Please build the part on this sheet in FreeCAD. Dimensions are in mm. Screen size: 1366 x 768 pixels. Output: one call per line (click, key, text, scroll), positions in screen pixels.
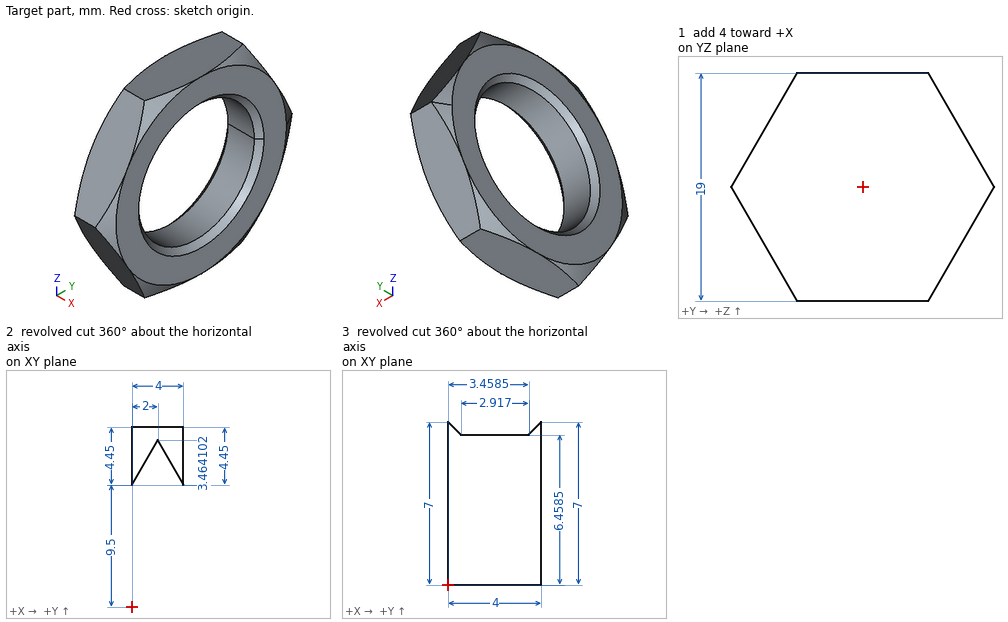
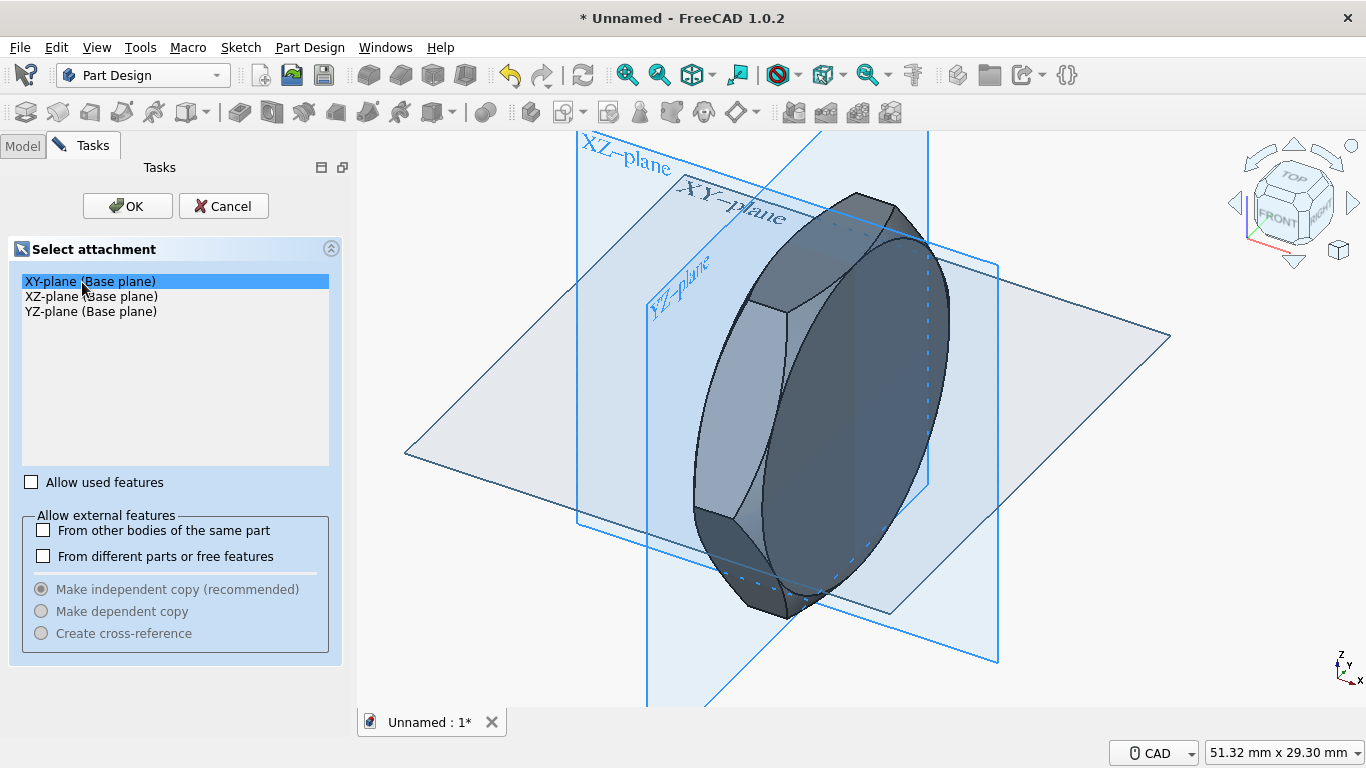
click(128, 206)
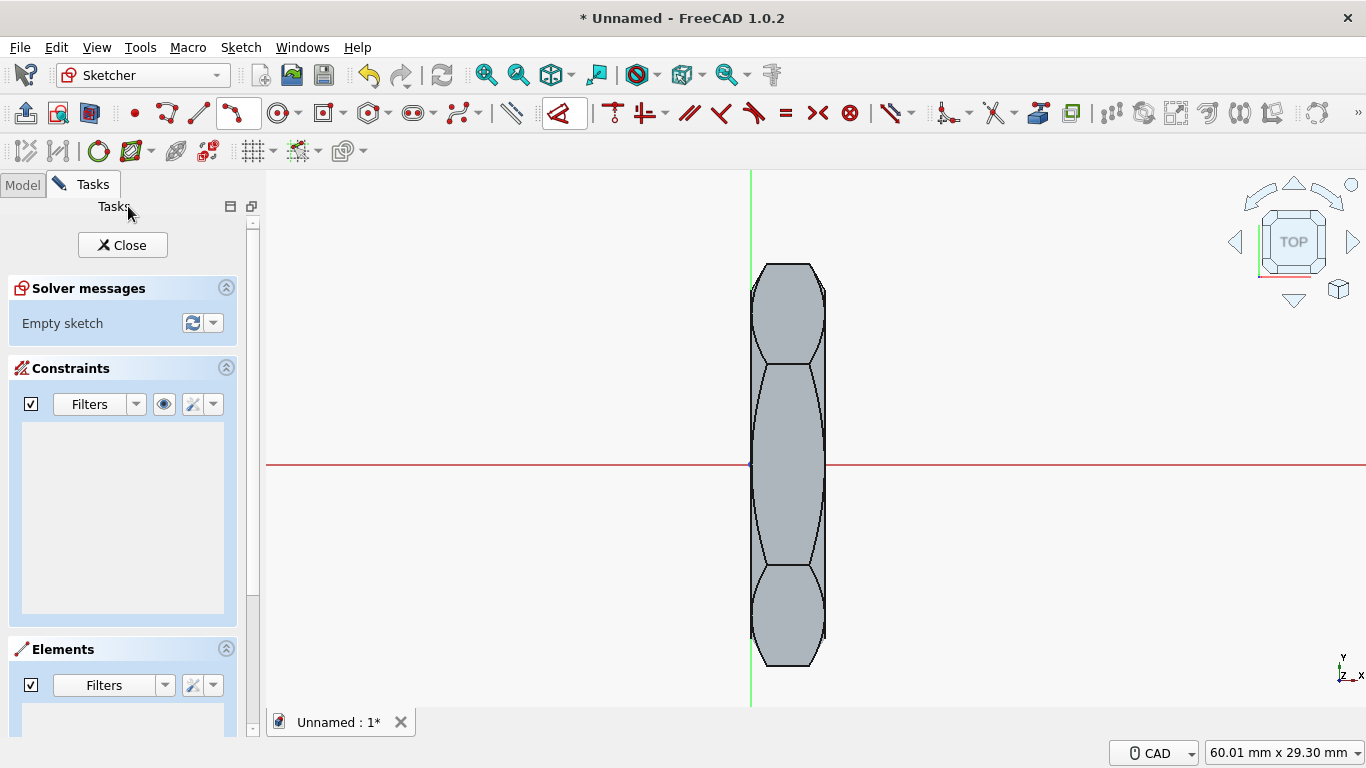
key(q)
key(s)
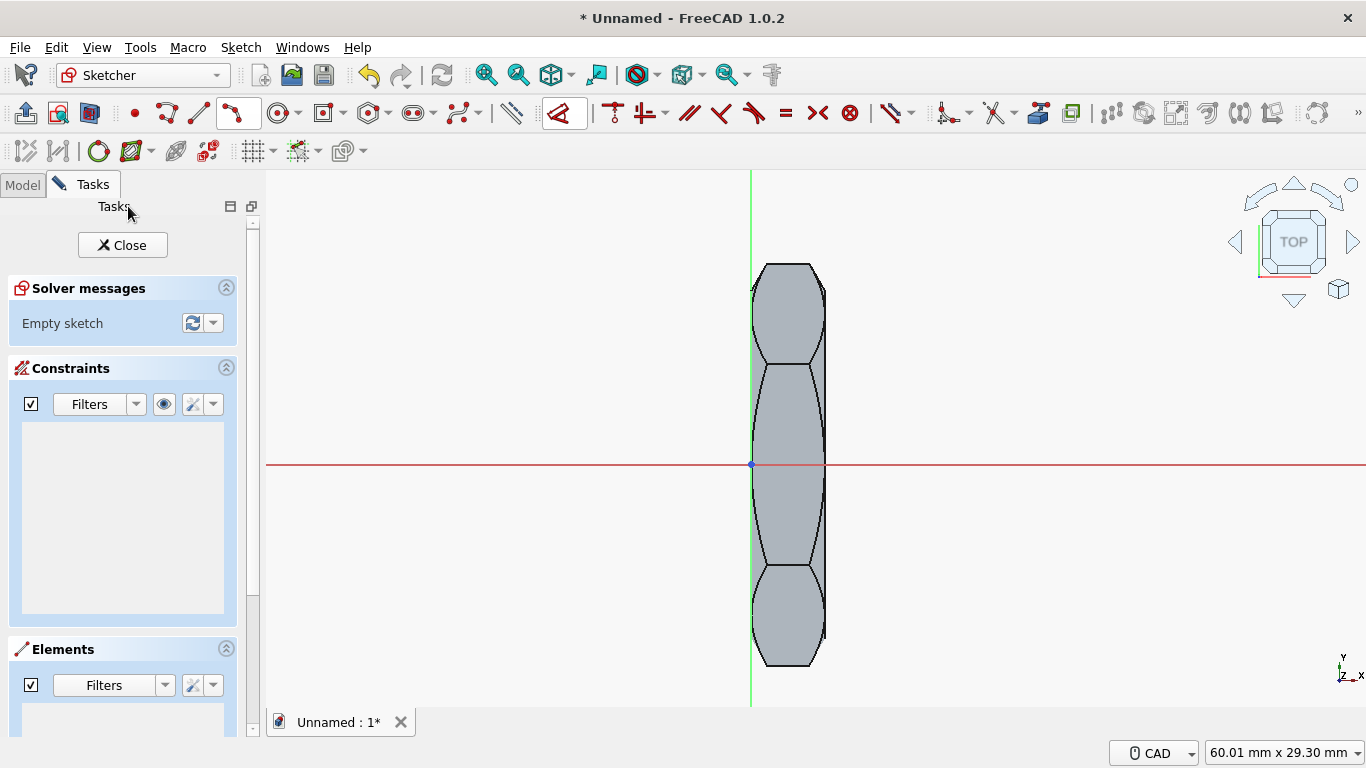
scroll(812, 378, up, 5)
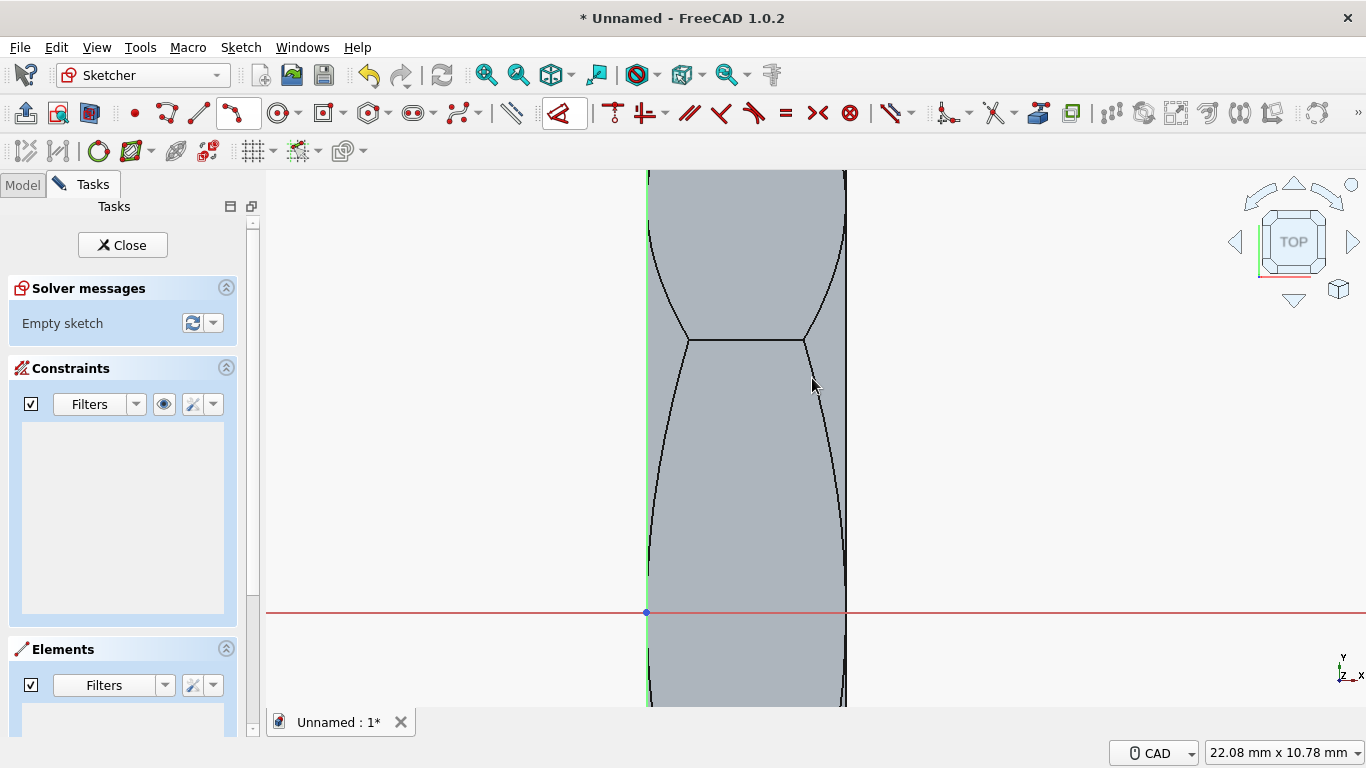
key(g)
key(m)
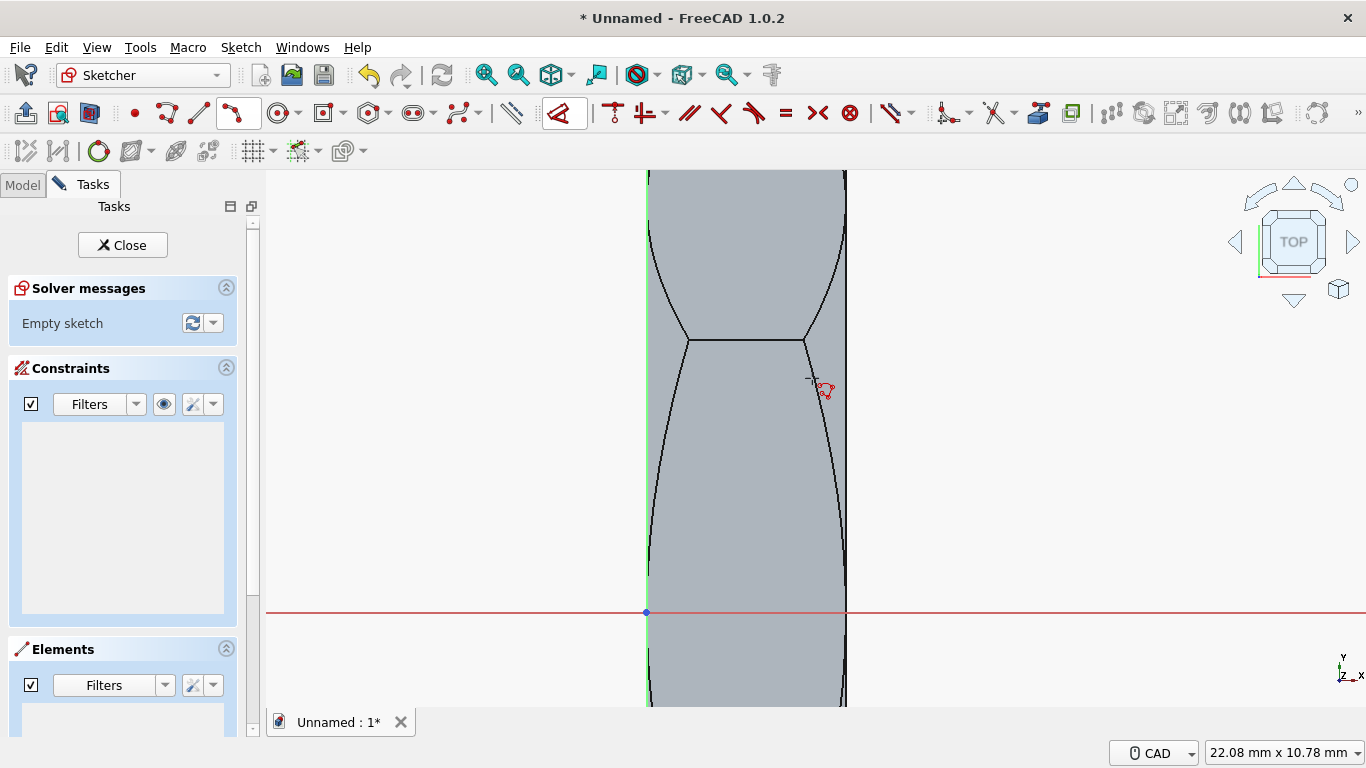
click(647, 613)
click(846, 604)
click(846, 264)
click(819, 291)
click(674, 291)
click(656, 264)
click(647, 613)
key(Escape)
key(Escape)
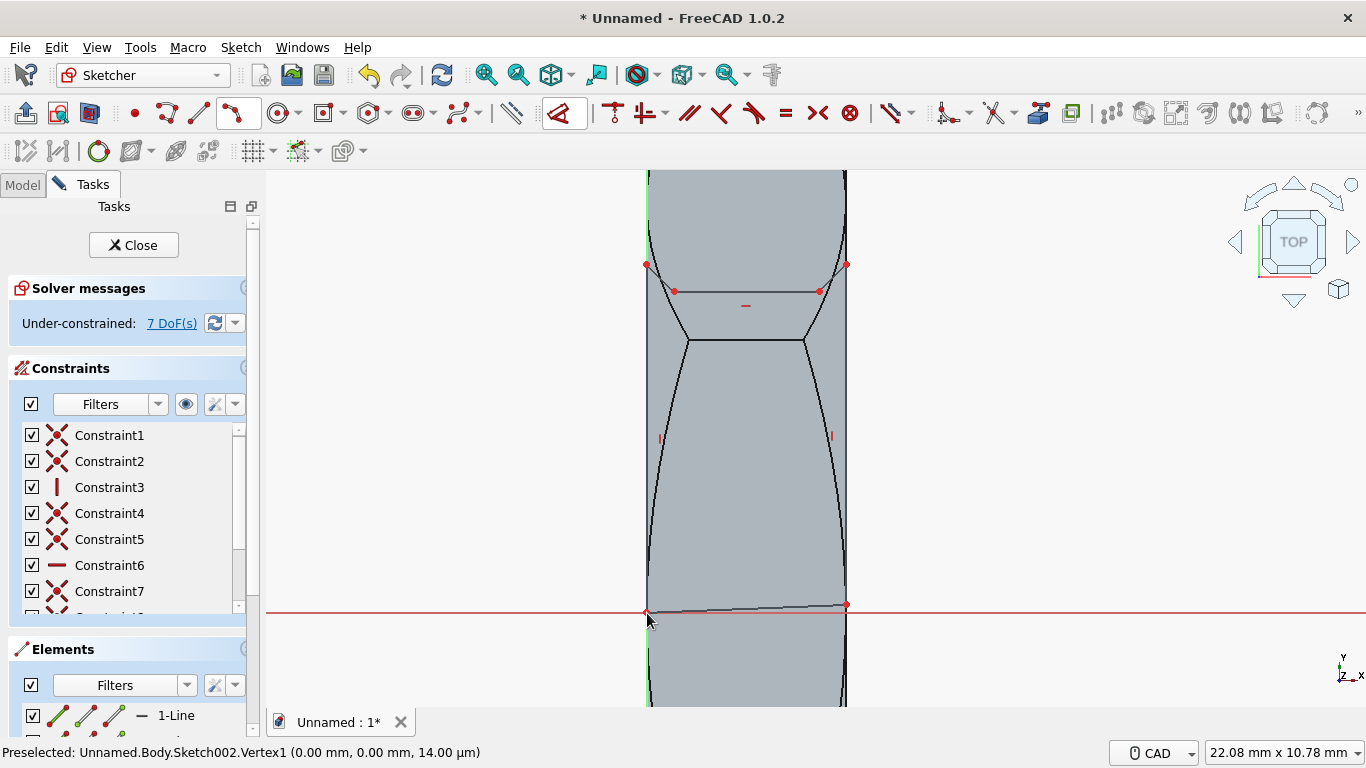
click(706, 611)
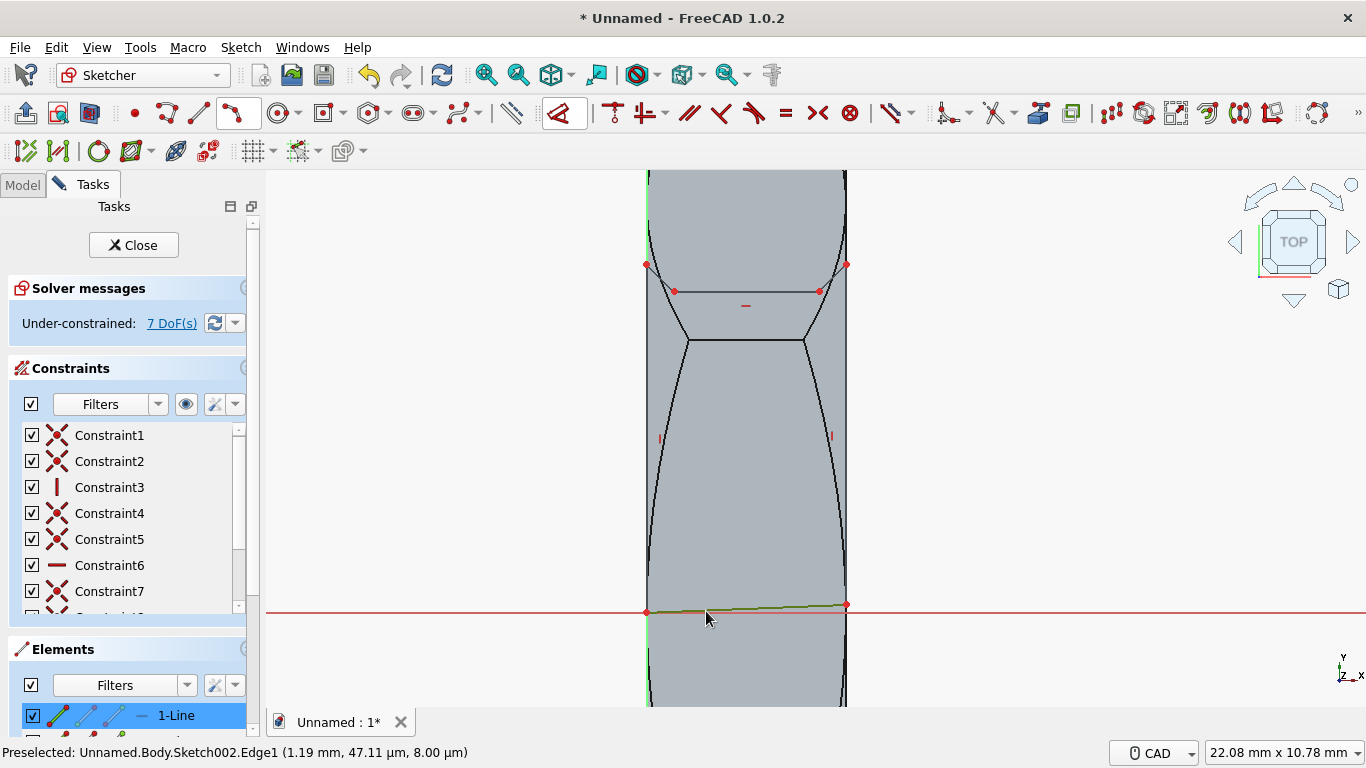
key(h)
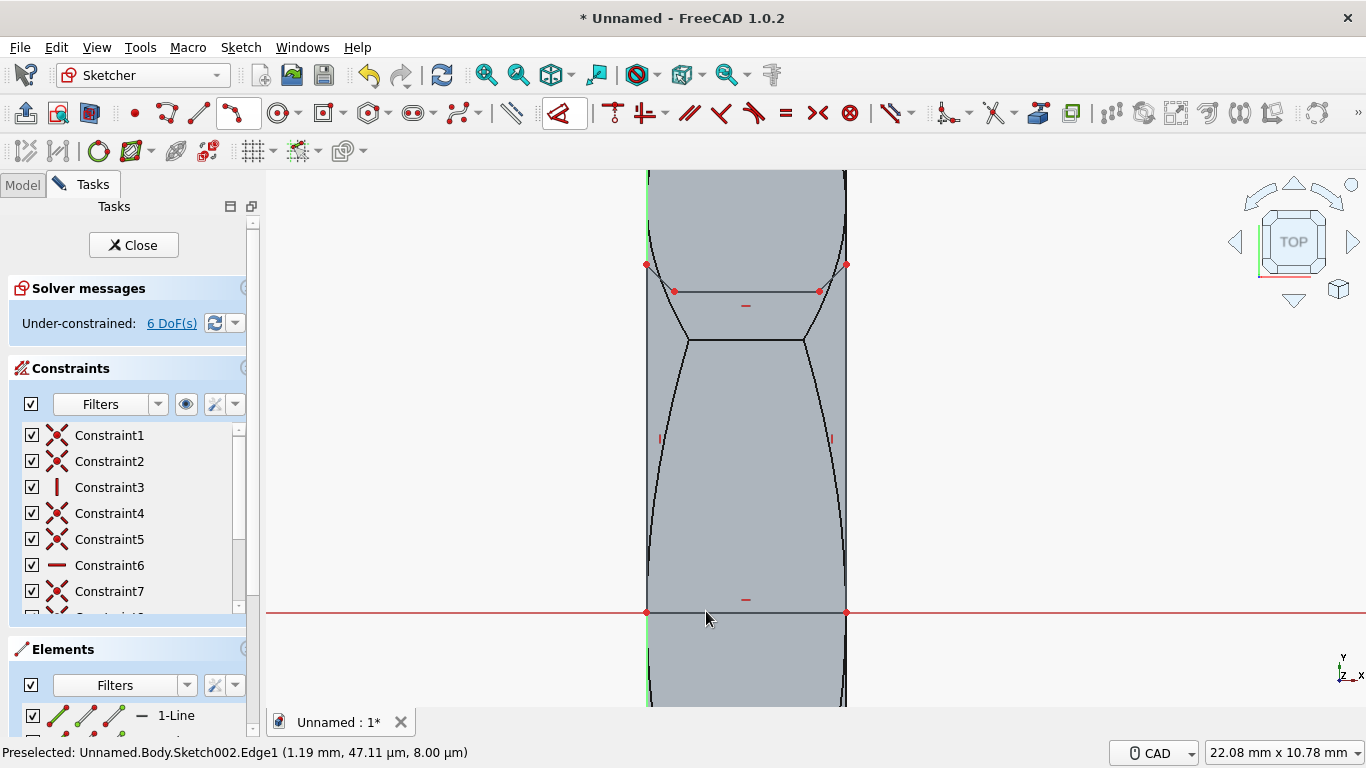
click(706, 613)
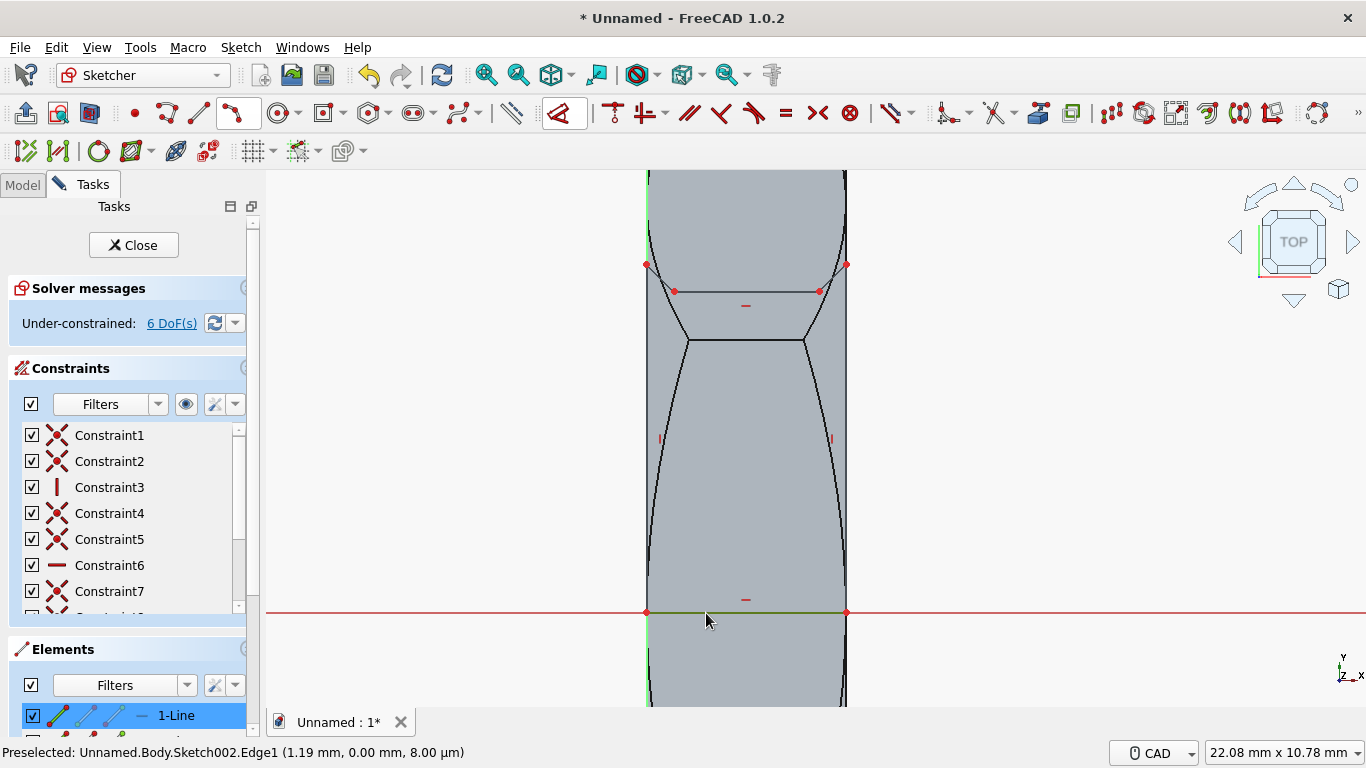
key(l)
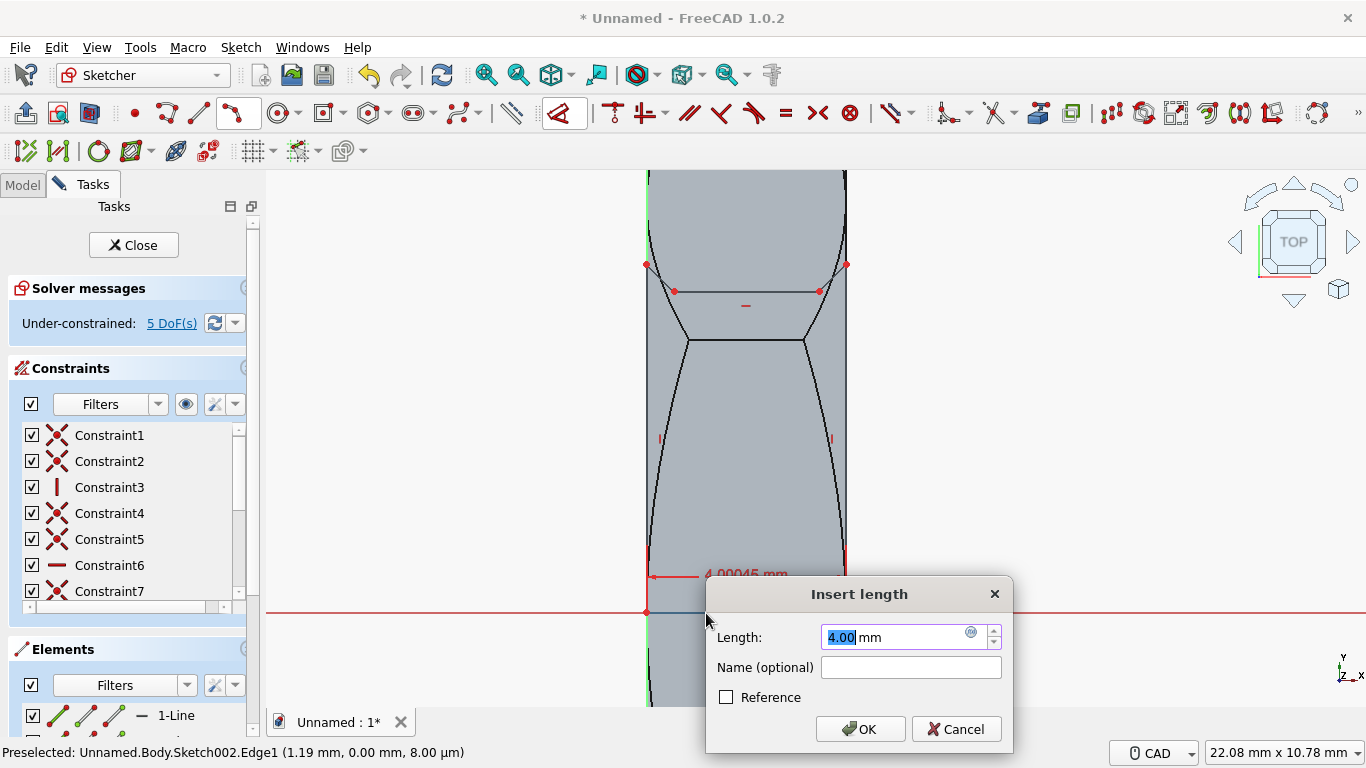
text(4)
key(Return)